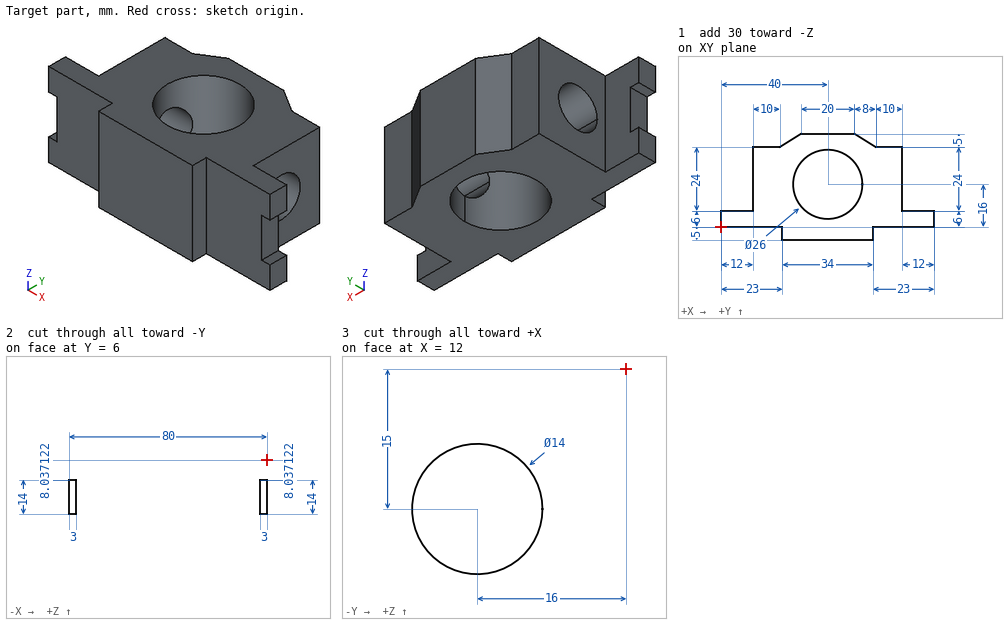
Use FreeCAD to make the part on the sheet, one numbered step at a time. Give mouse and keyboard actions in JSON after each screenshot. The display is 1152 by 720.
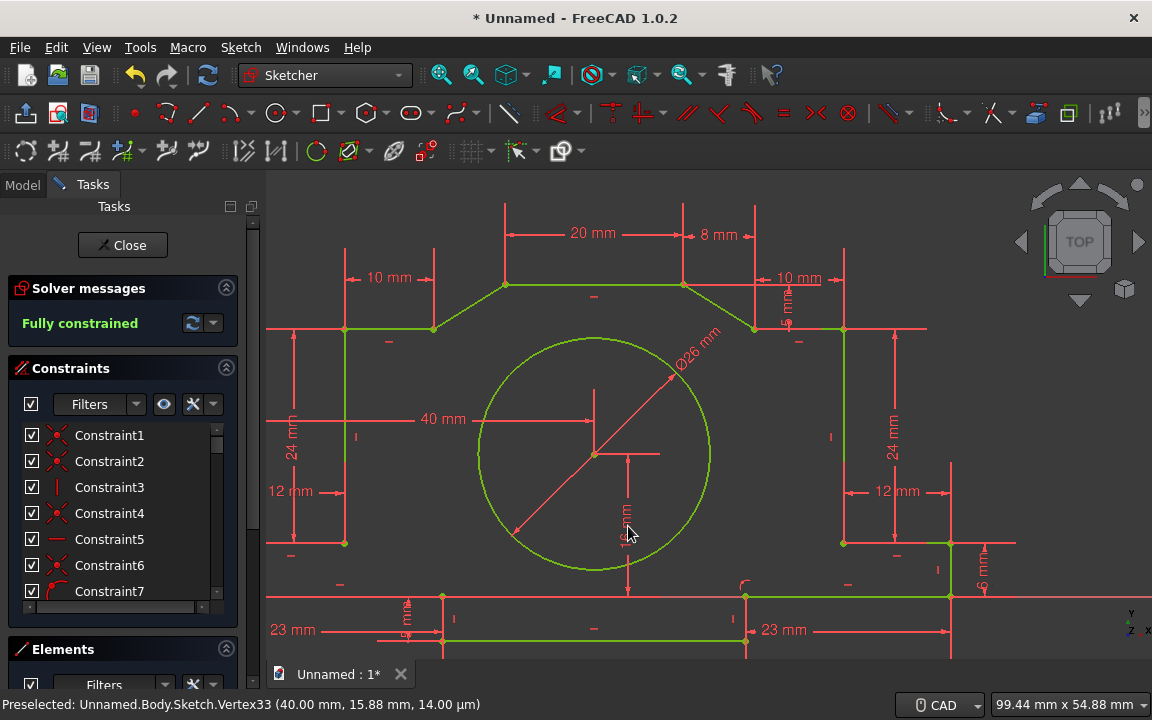
{"action": "left_click", "coordinate": [123, 245]}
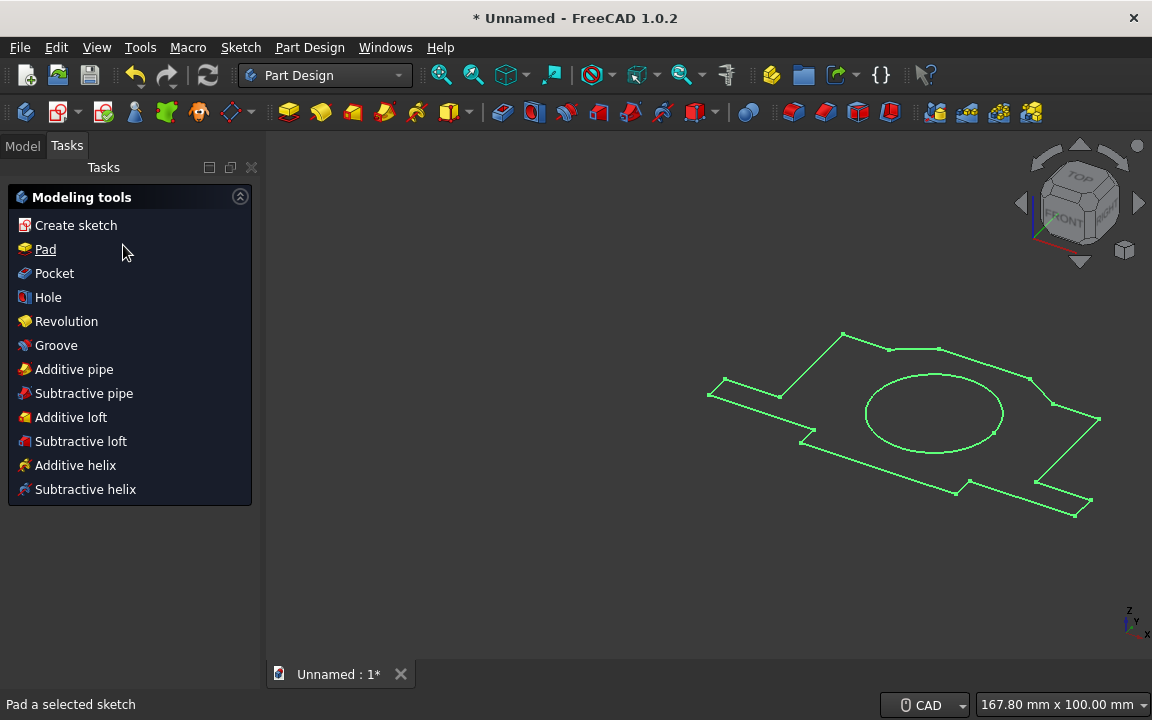
{"action": "left_click", "coordinate": [290, 112]}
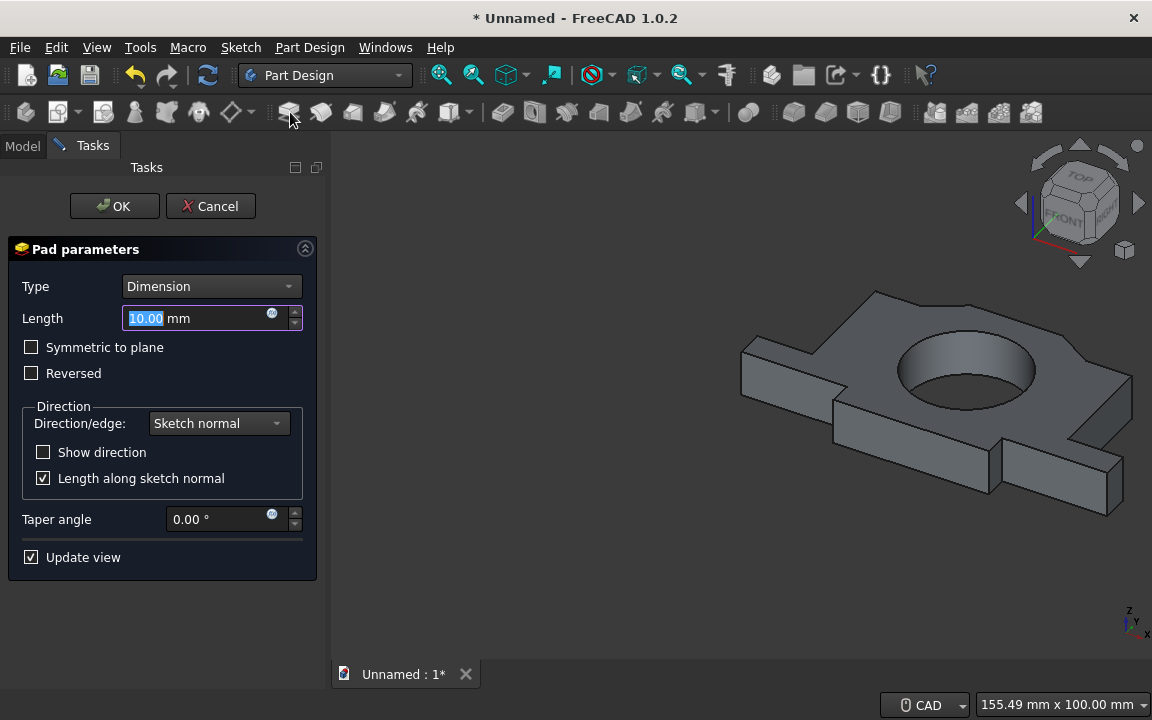
{"action": "type", "text": "30"}
{"action": "key", "text": "Tab"}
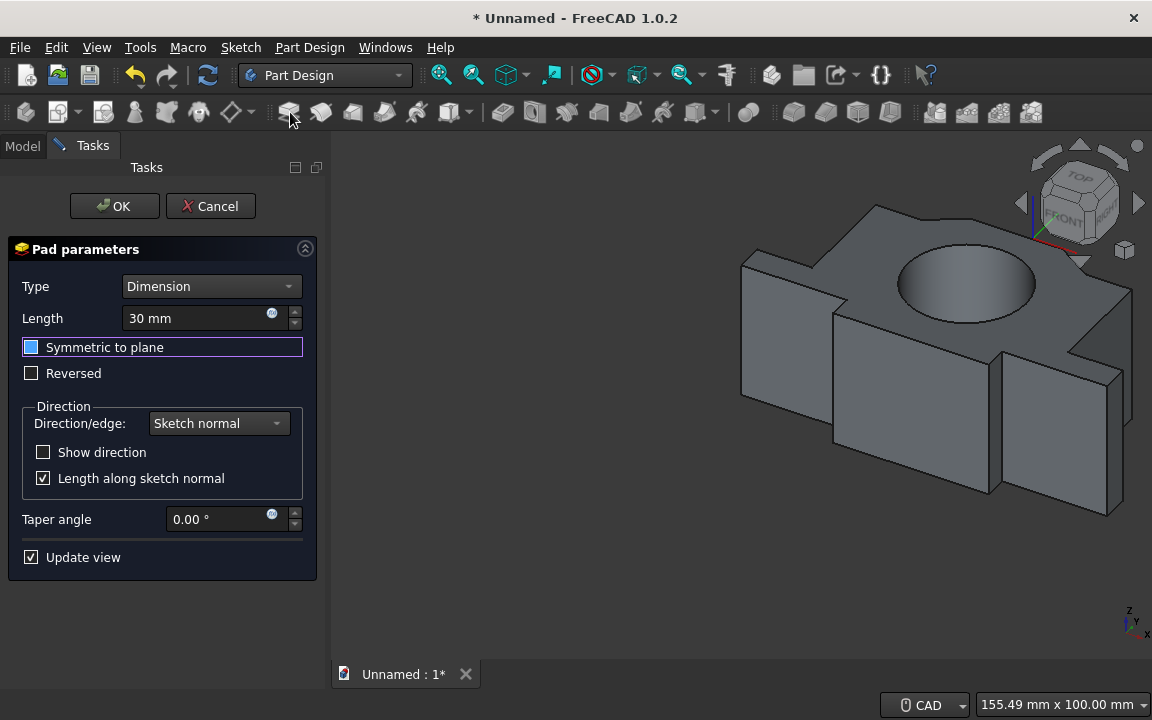
{"action": "left_click", "coordinate": [30, 373]}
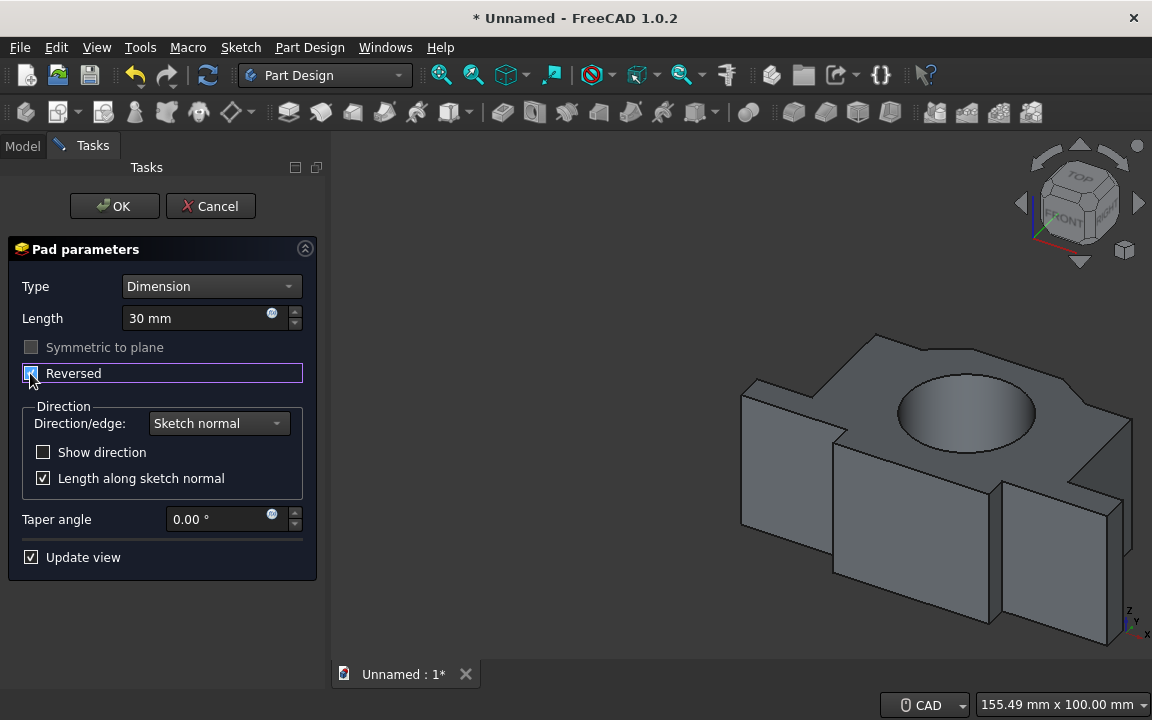
{"action": "left_click", "coordinate": [115, 206]}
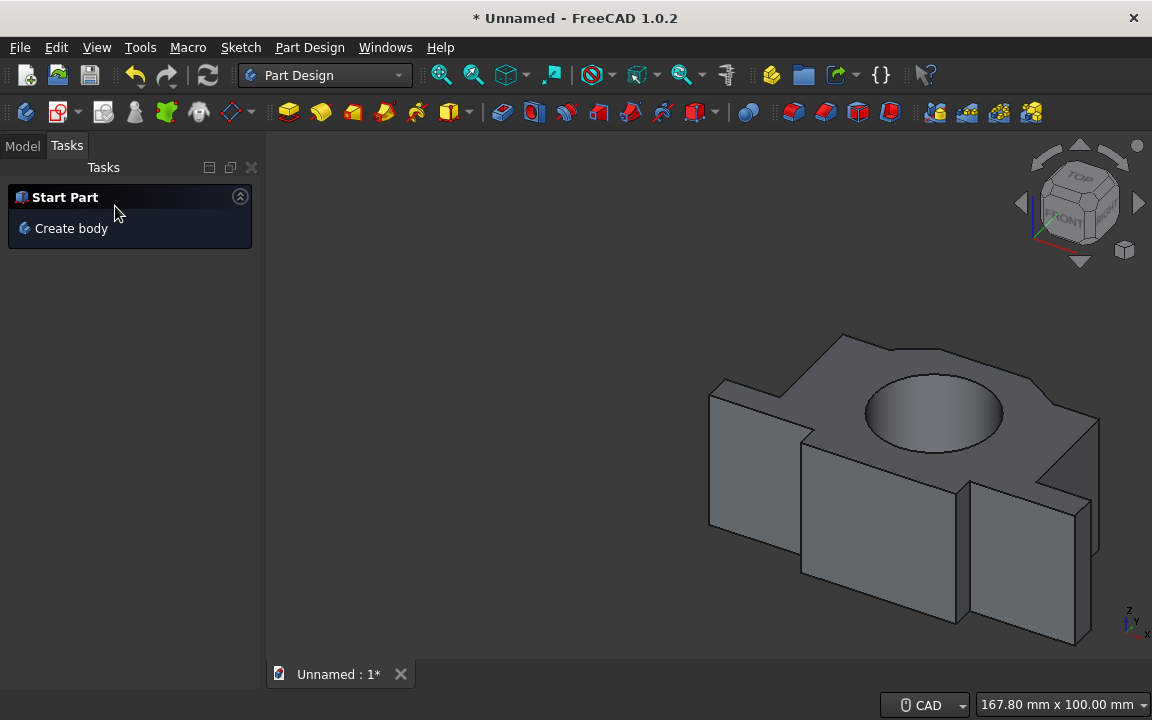
{"action": "key", "text": "v f"}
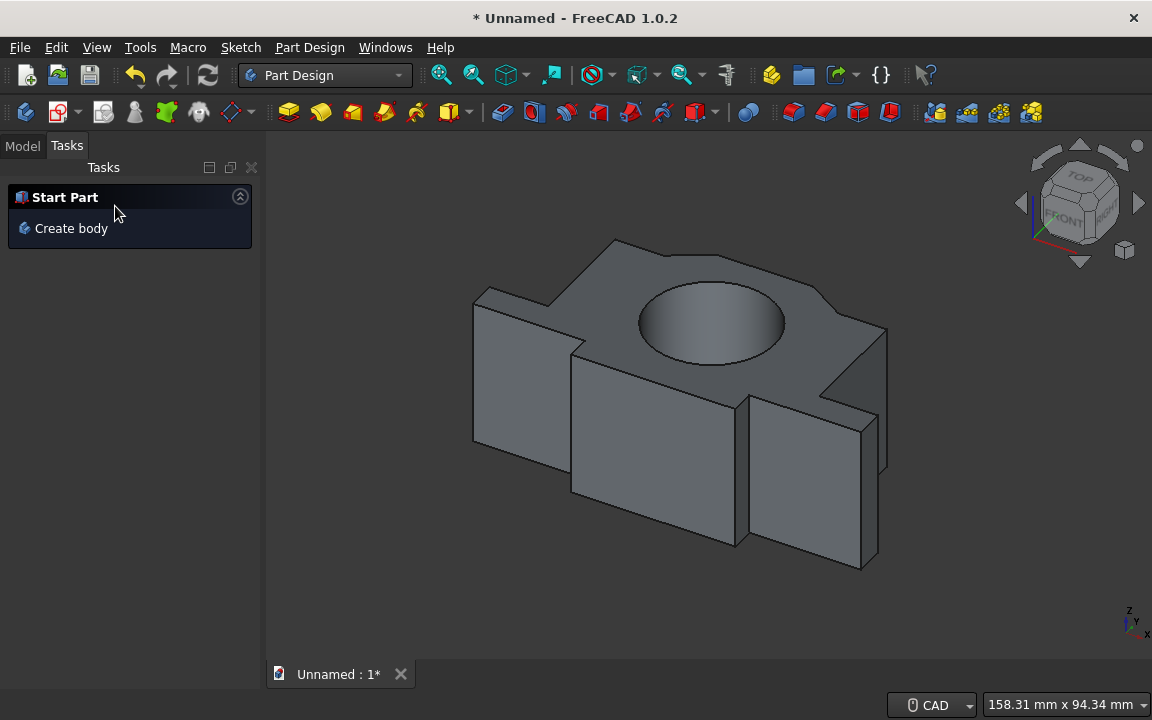
{"action": "key", "text": "4"}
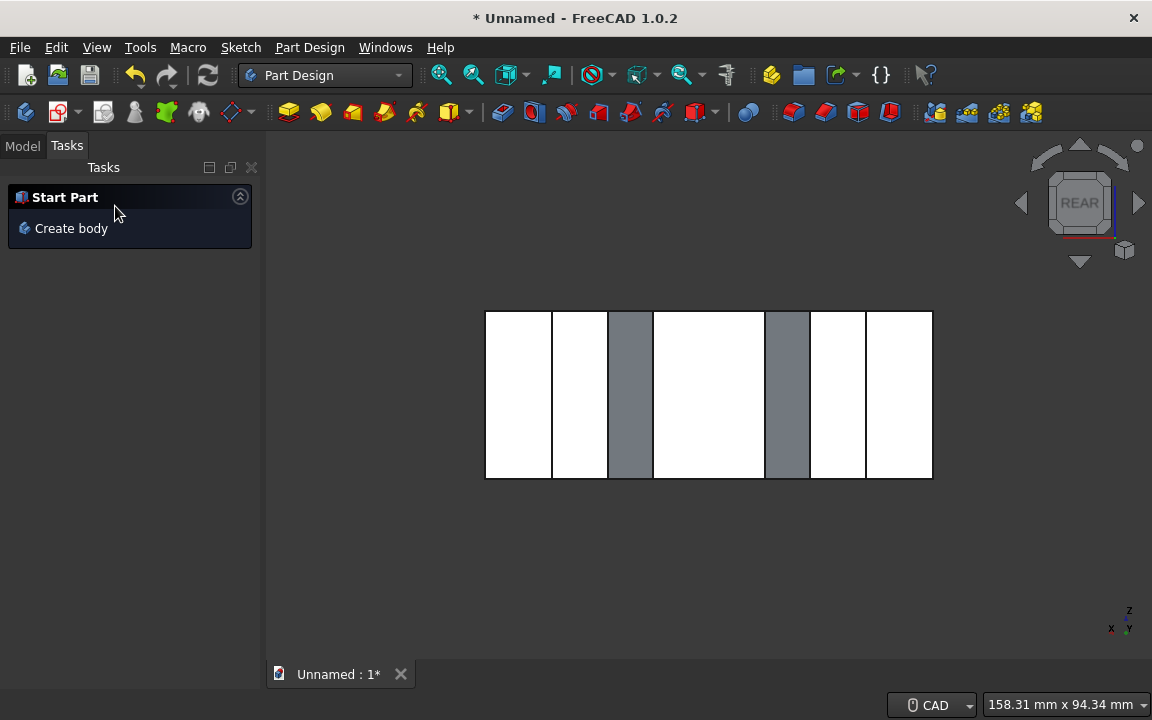
{"action": "left_click", "coordinate": [519, 346]}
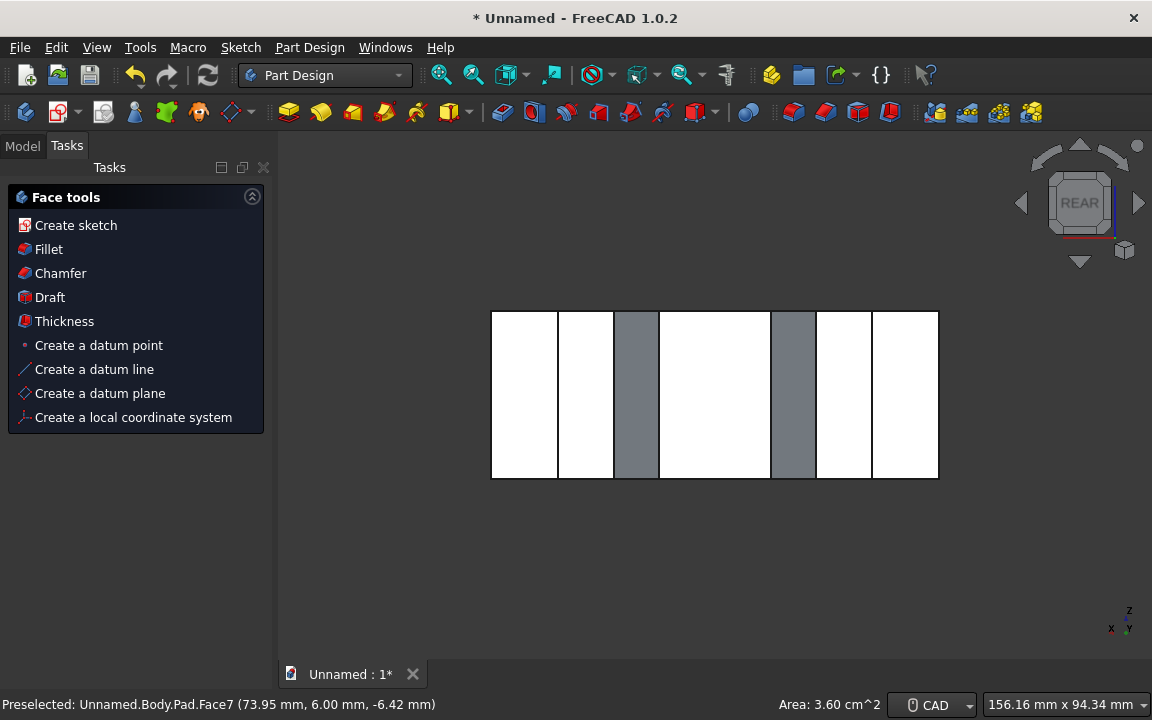
{"action": "left_click", "coordinate": [58, 112]}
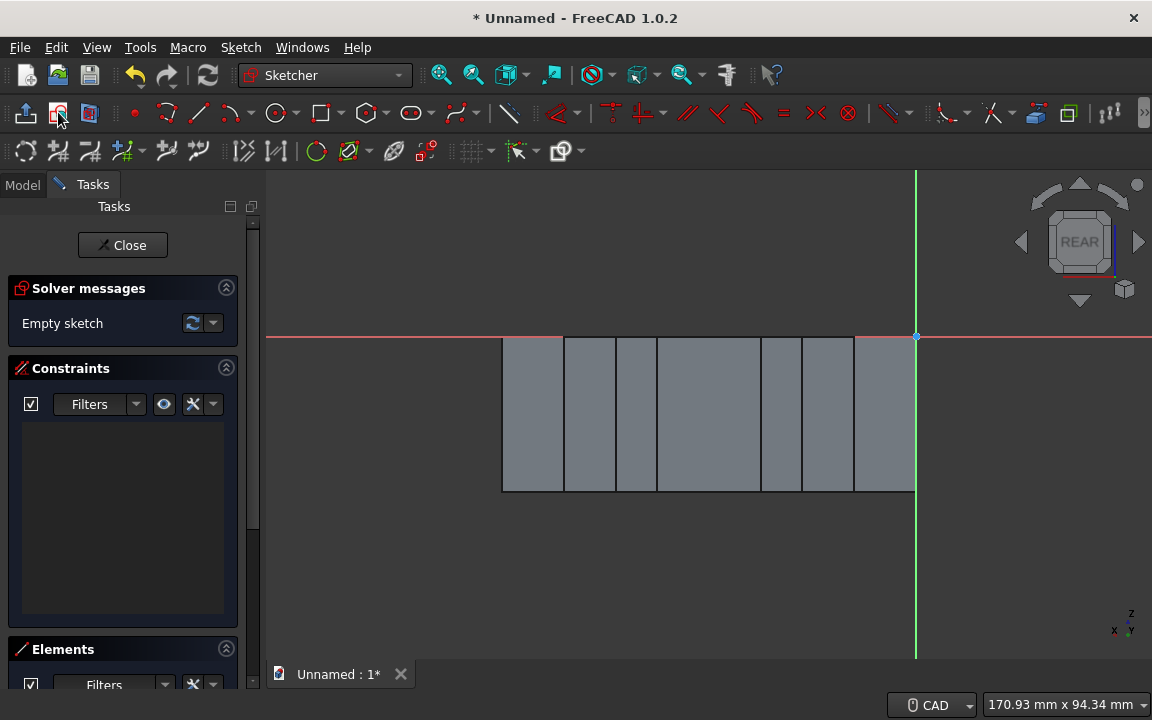
{"action": "key", "text": "g r"}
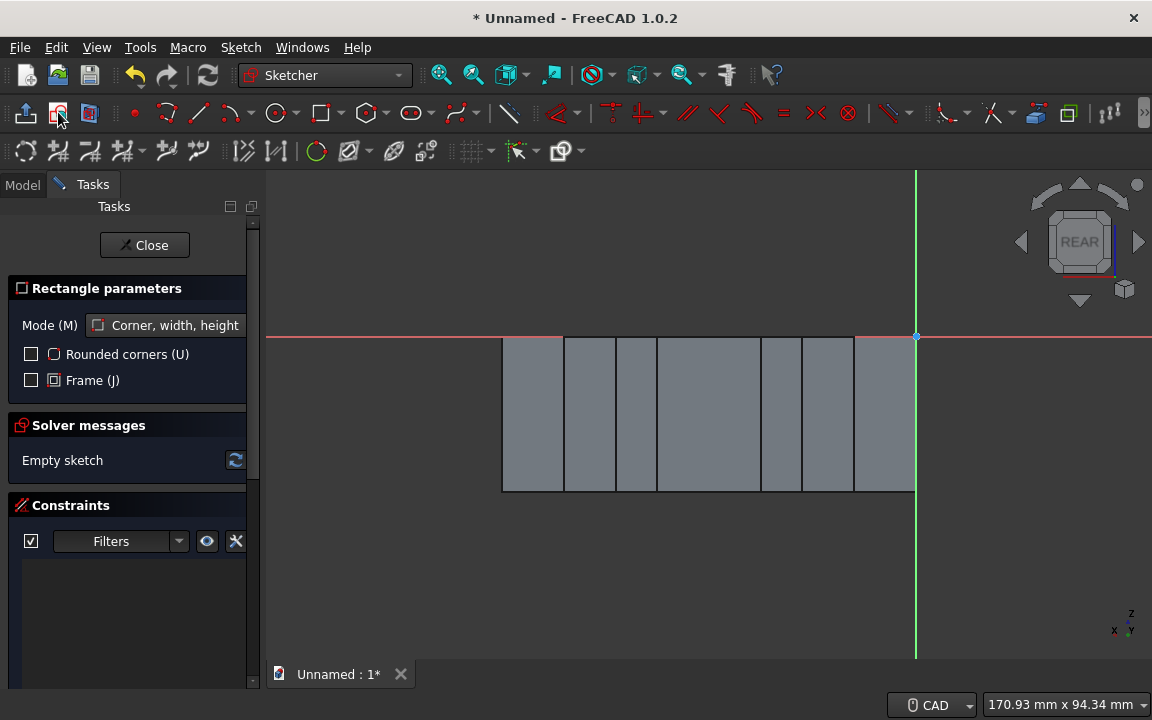
{"action": "left_click", "coordinate": [901, 378]}
{"action": "left_click", "coordinate": [916, 451]}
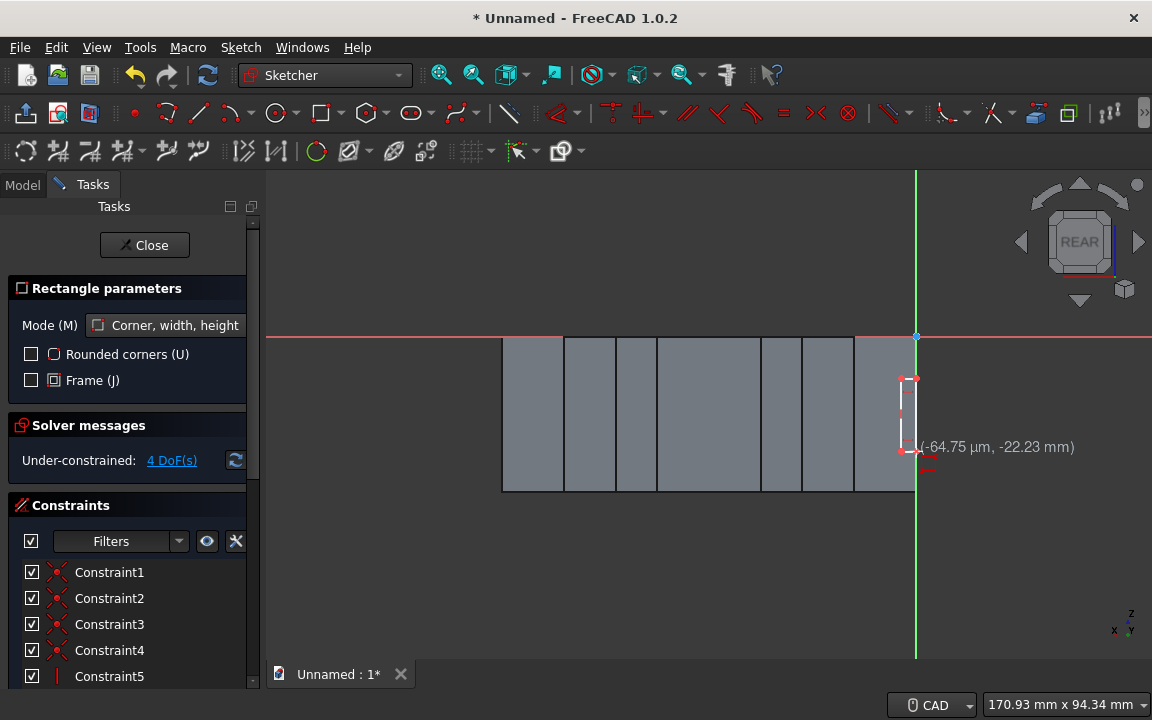
{"action": "left_click", "coordinate": [502, 378]}
{"action": "left_click", "coordinate": [517, 451]}
{"action": "key", "text": "Escape"}